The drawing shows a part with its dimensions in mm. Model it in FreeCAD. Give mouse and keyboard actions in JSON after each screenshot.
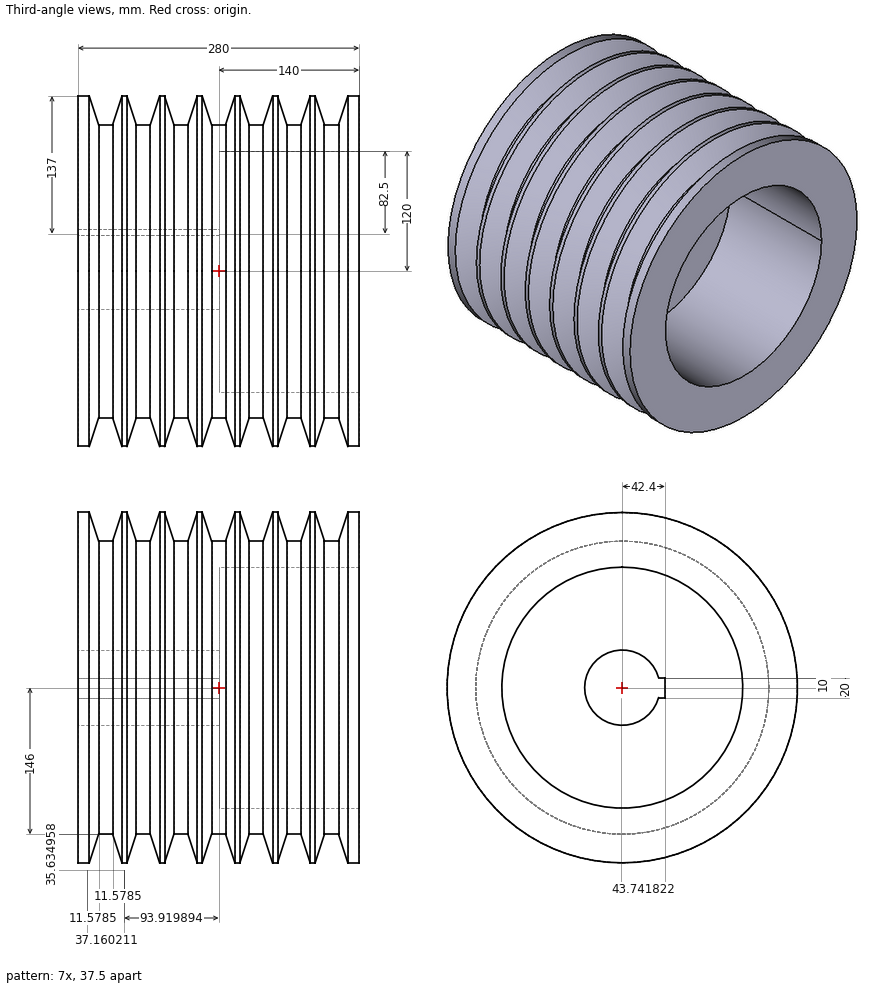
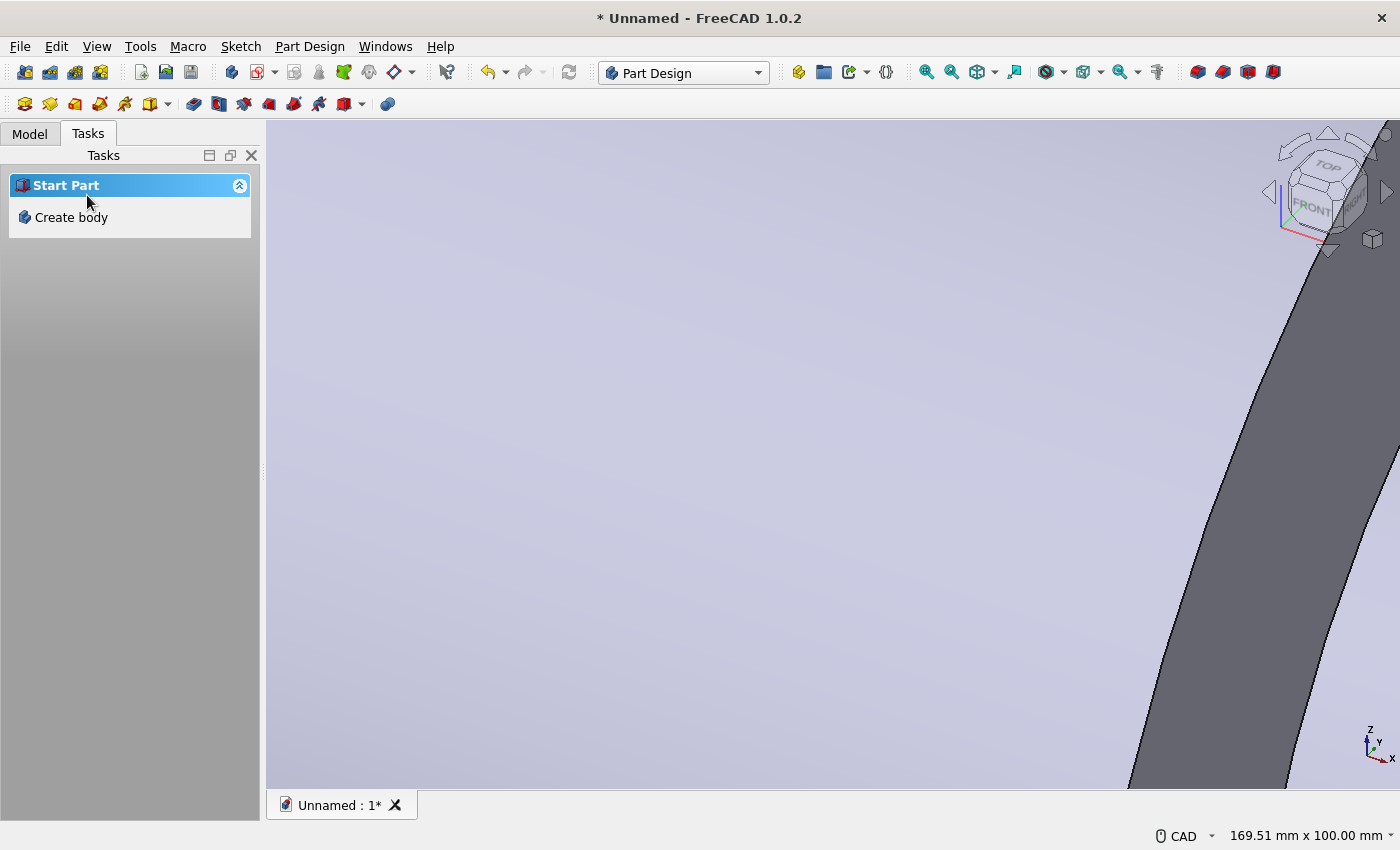
{"action": "left_click", "coordinate": [927, 72]}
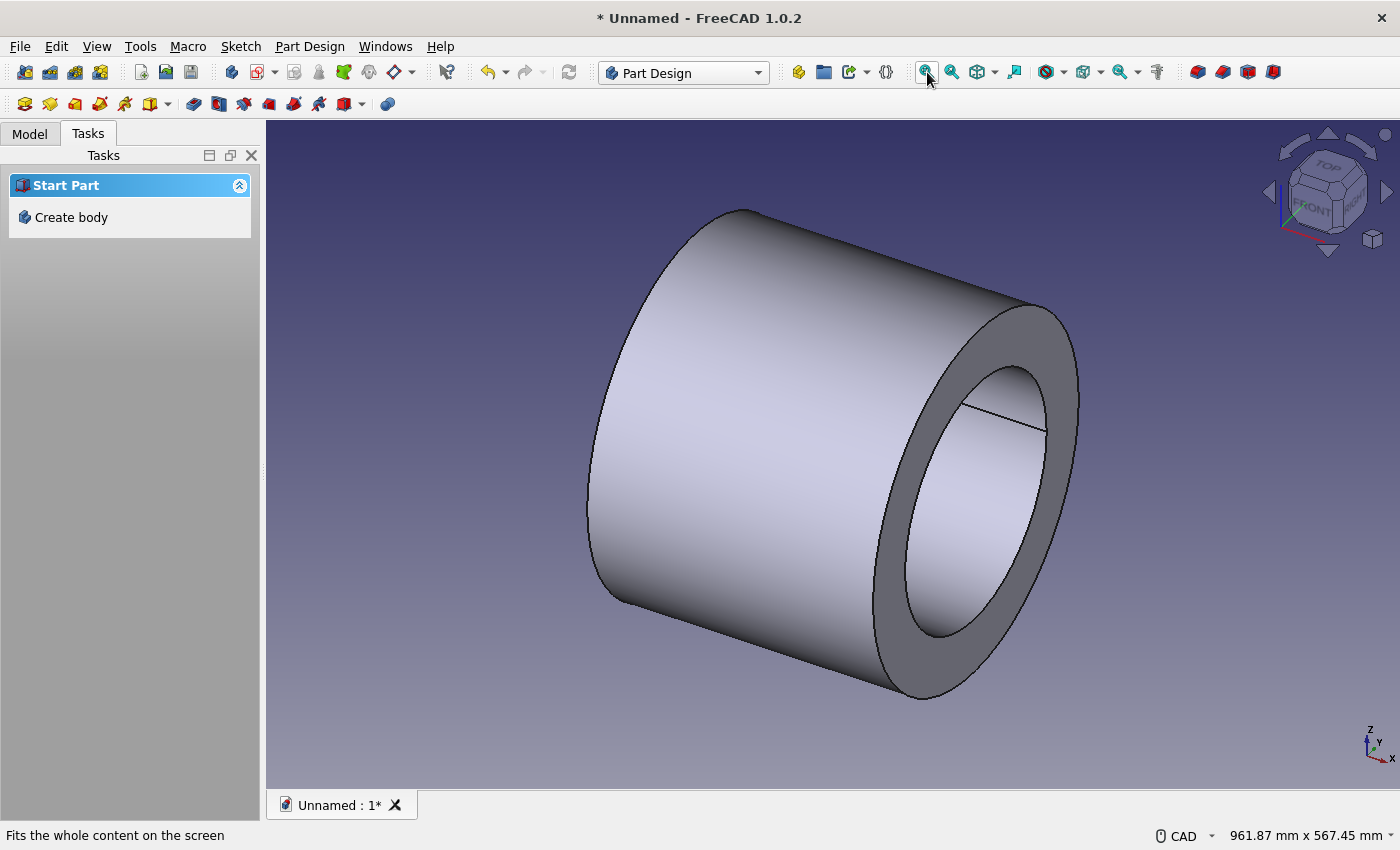
{"action": "left_click", "coordinate": [256, 72]}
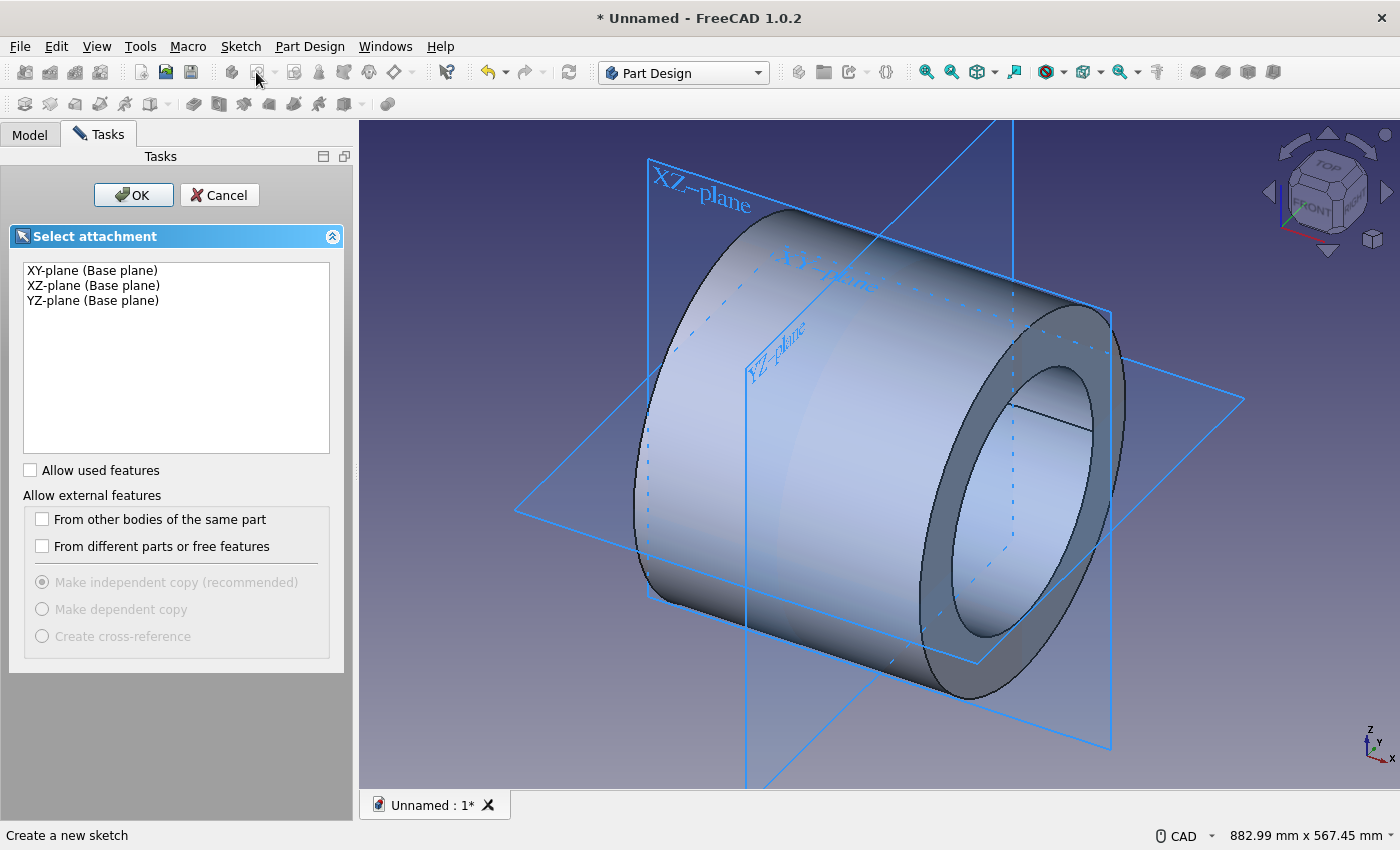
{"action": "left_click", "coordinate": [84, 286]}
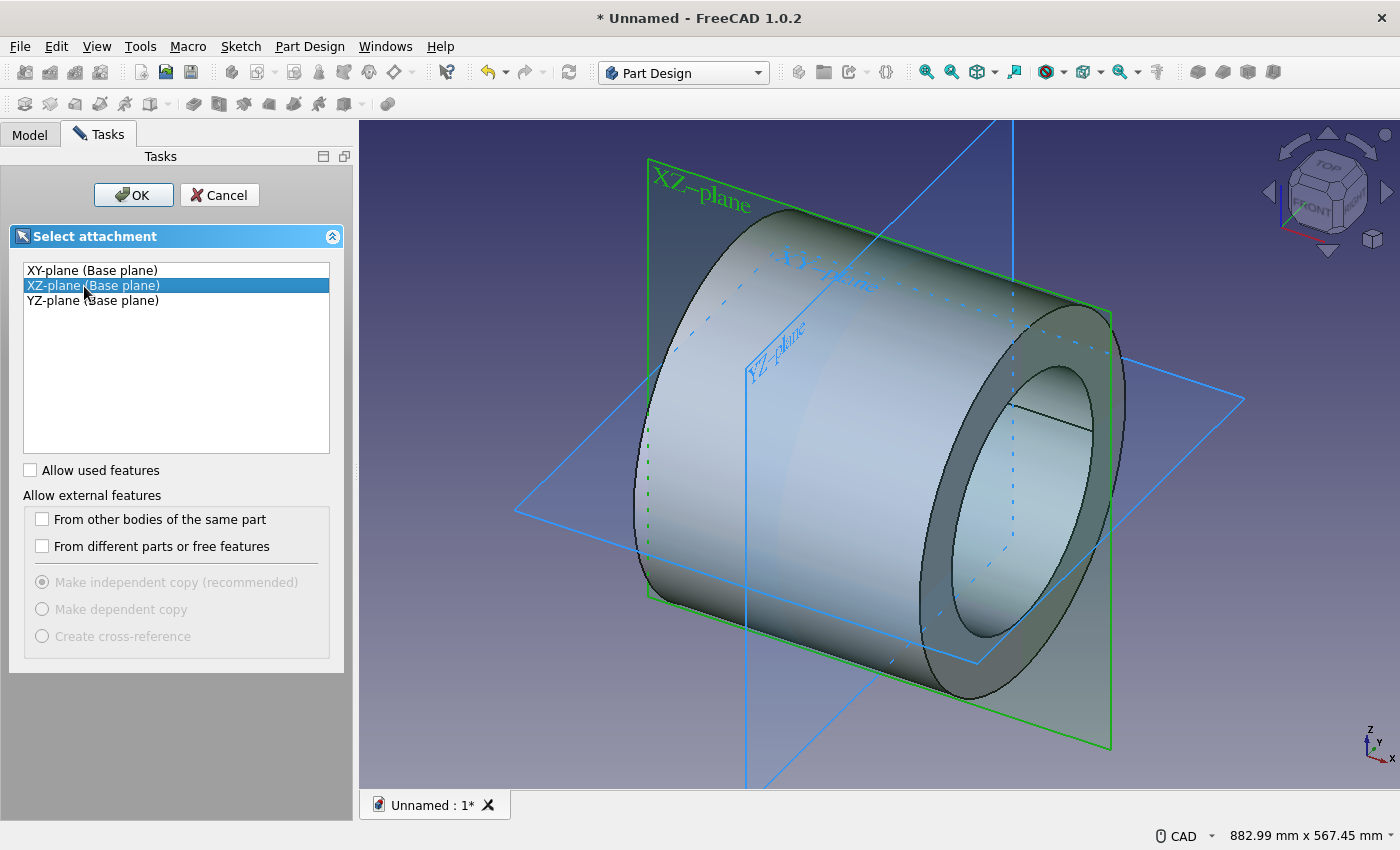
{"action": "left_click", "coordinate": [134, 195]}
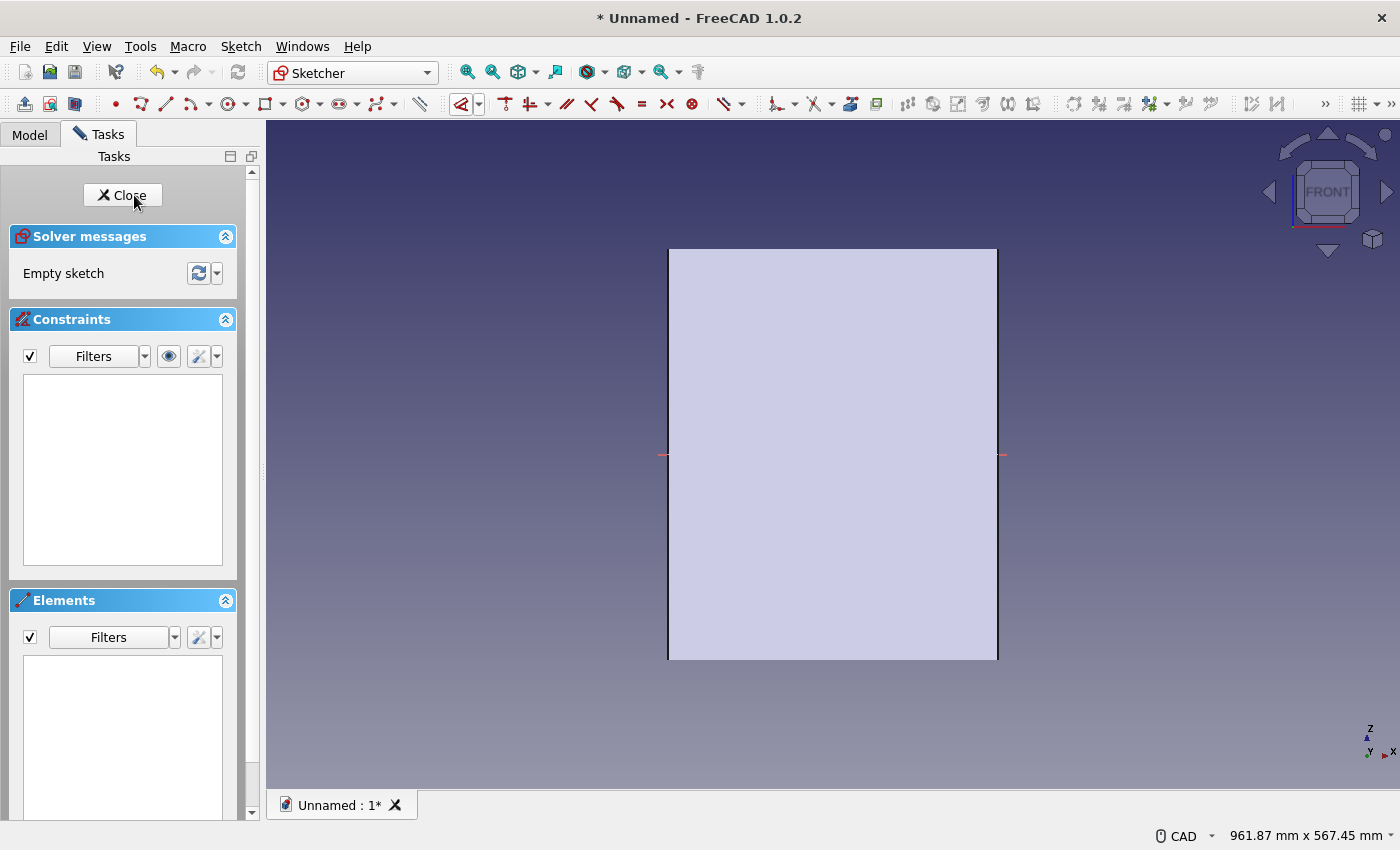
{"action": "left_click", "coordinate": [75, 104]}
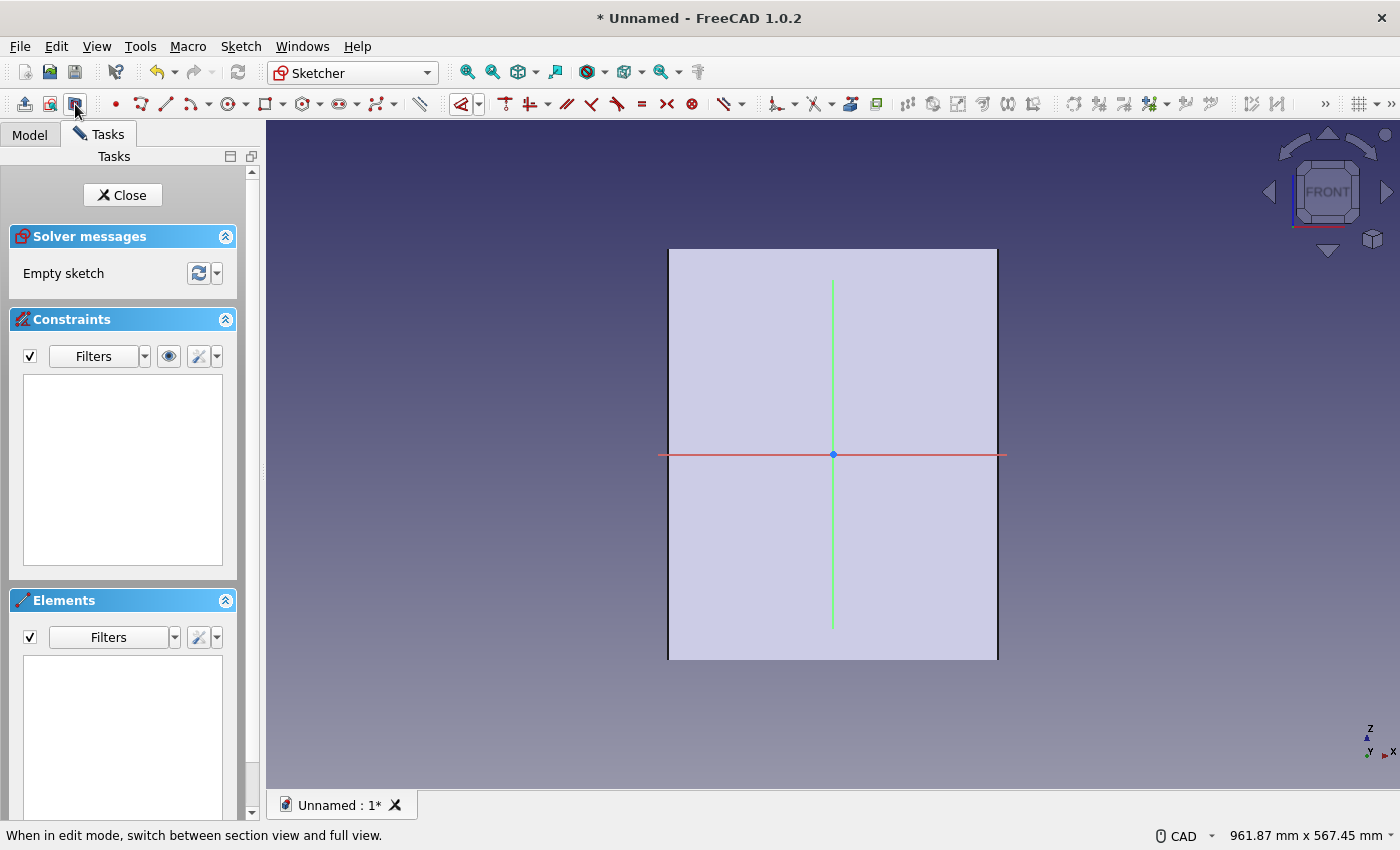
{"action": "scroll", "coordinate": [694, 667], "scroll_direction": "up", "scroll_amount": 12}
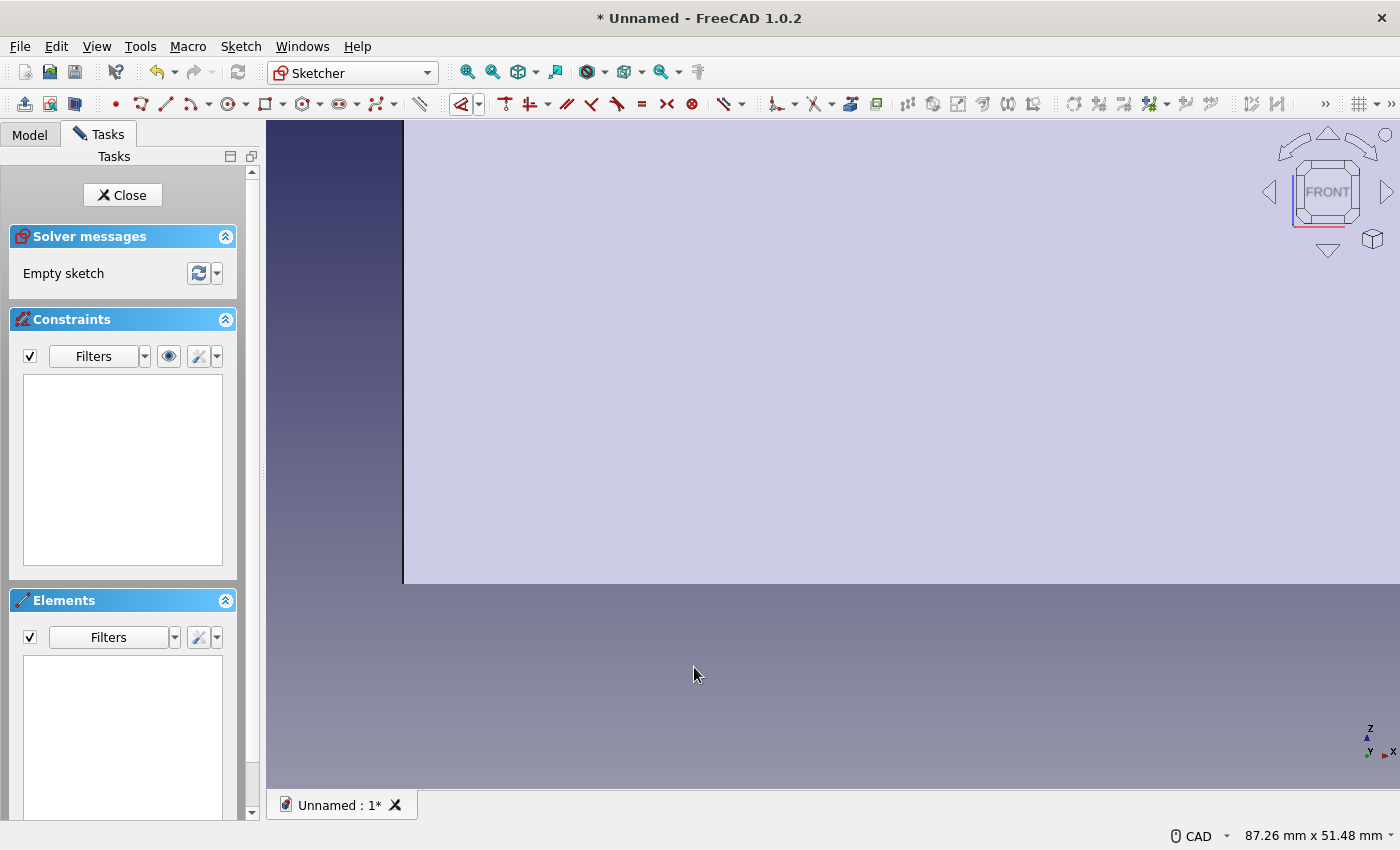
{"action": "left_click", "coordinate": [141, 104]}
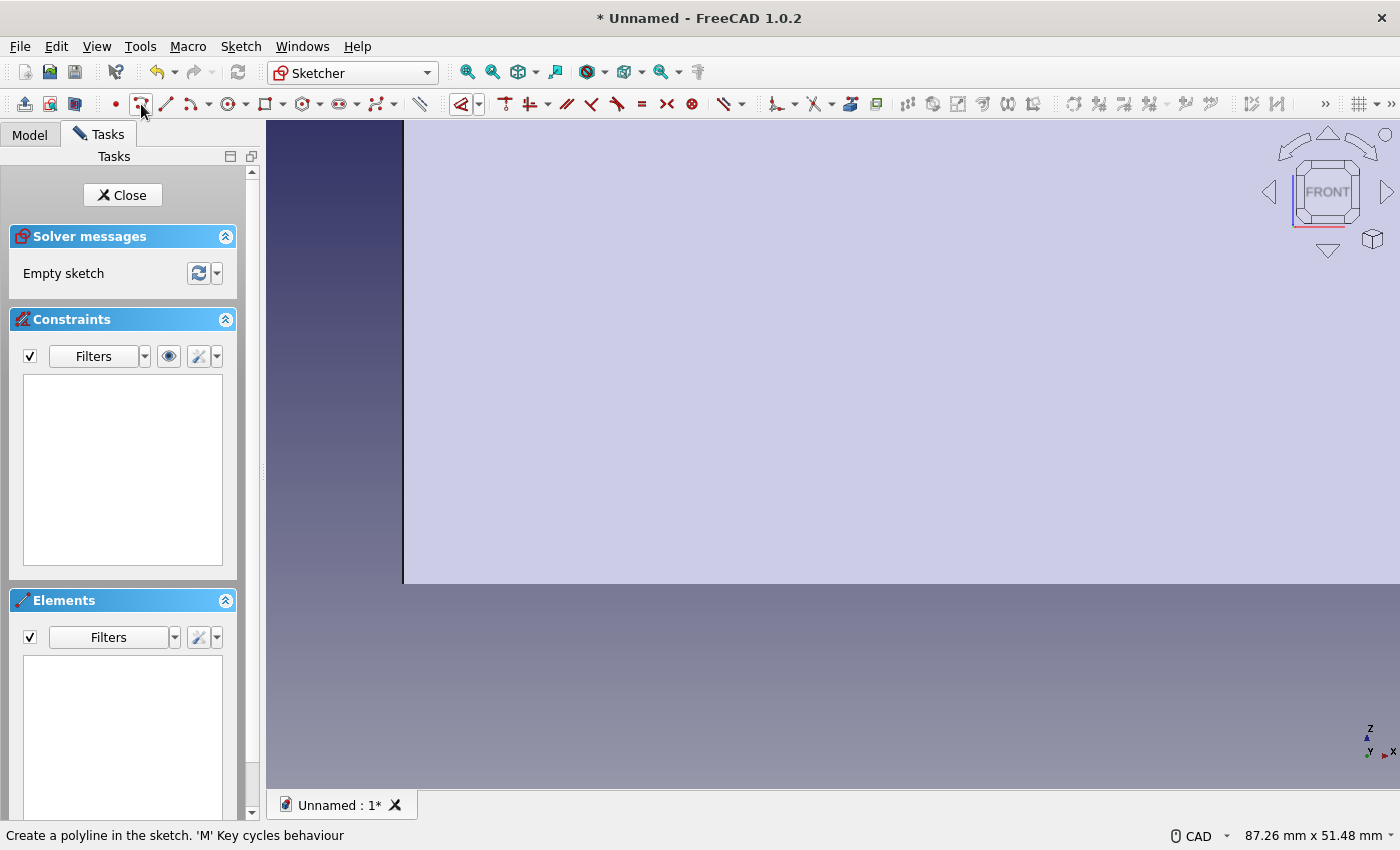
{"action": "left_click", "coordinate": [851, 214]}
{"action": "left_click", "coordinate": [1002, 677]}
{"action": "left_click", "coordinate": [519, 677]}
{"action": "left_click", "coordinate": [669, 214]}
{"action": "left_click", "coordinate": [851, 215]}
{"action": "key", "text": "Escape"}
{"action": "key", "text": "Escape"}